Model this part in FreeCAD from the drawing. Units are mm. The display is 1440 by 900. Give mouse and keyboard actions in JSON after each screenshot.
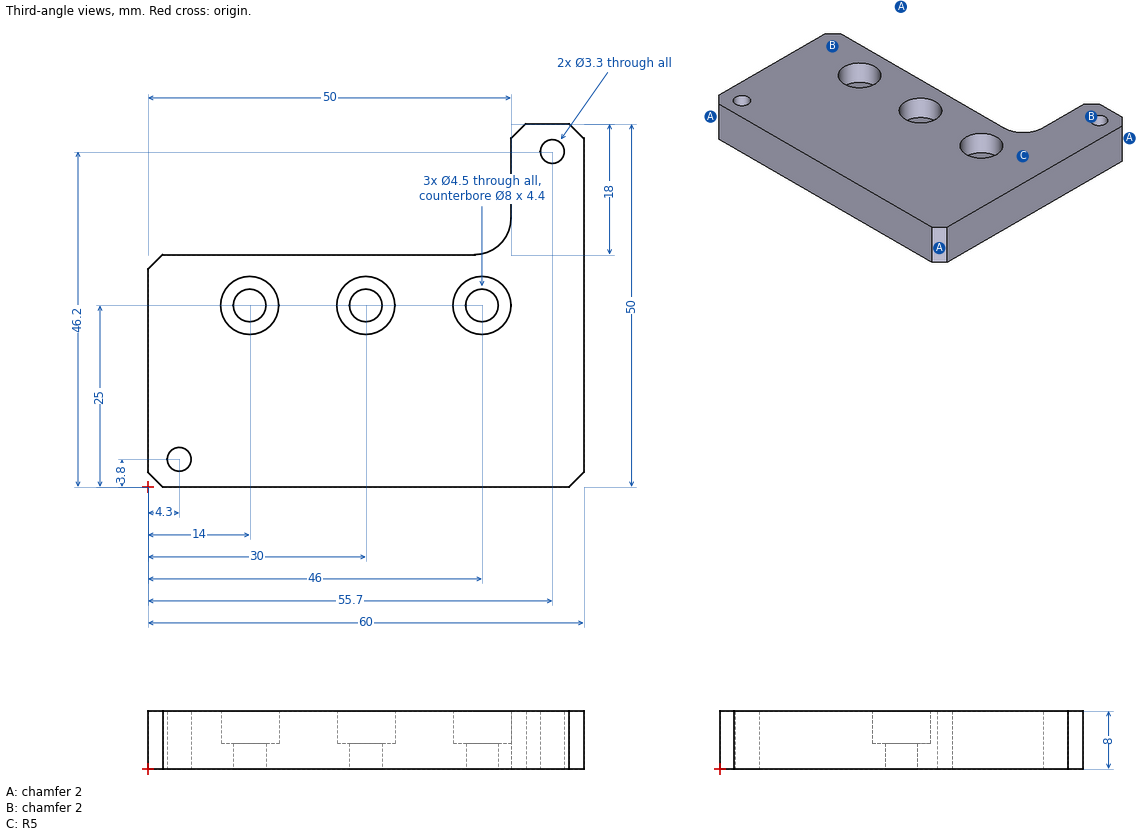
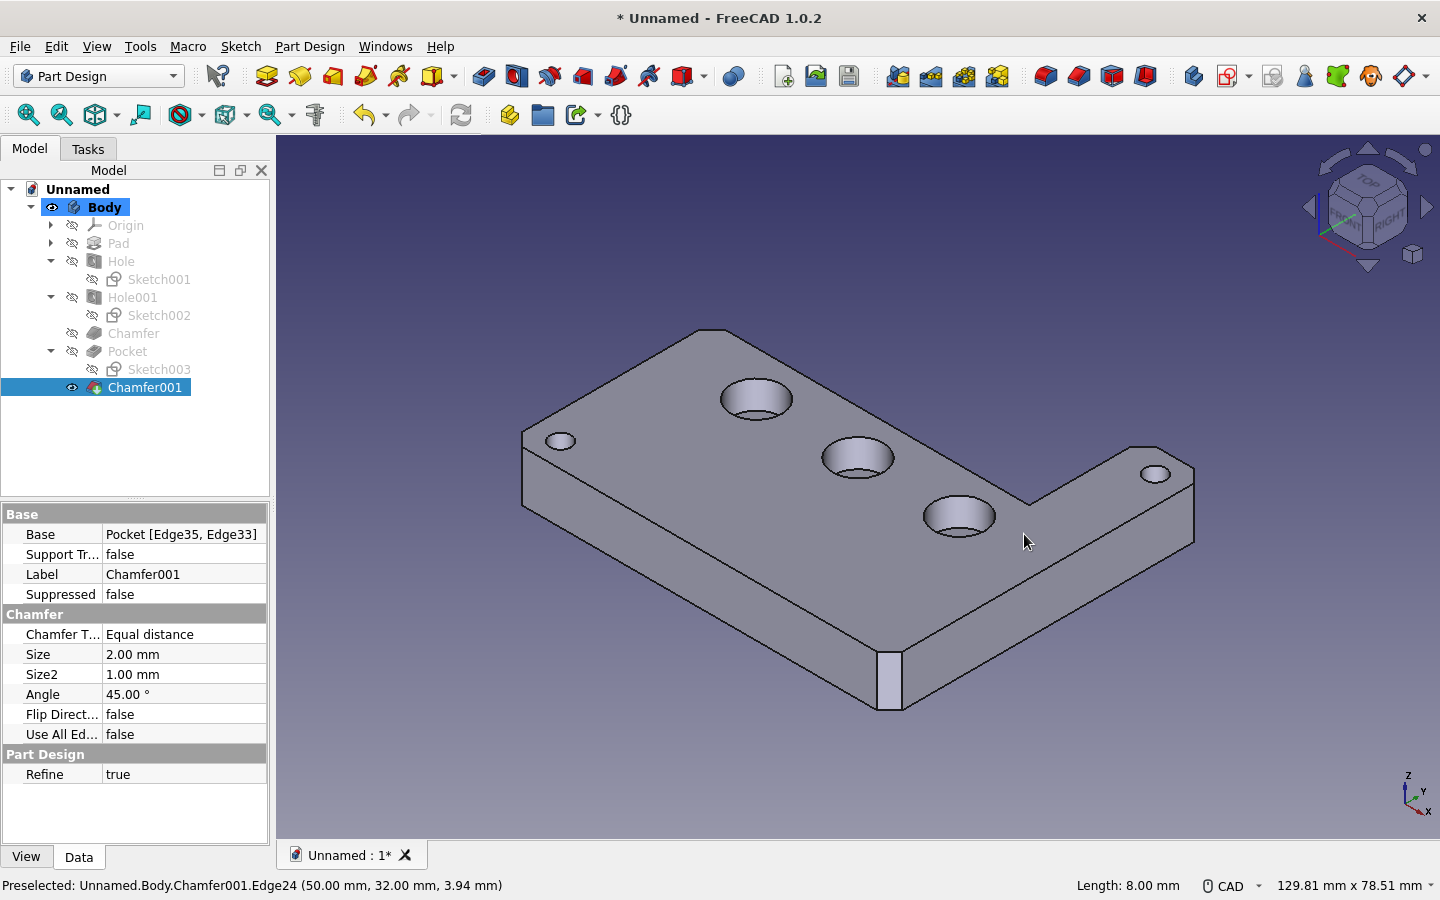
{"action": "left_click", "coordinate": [1046, 76]}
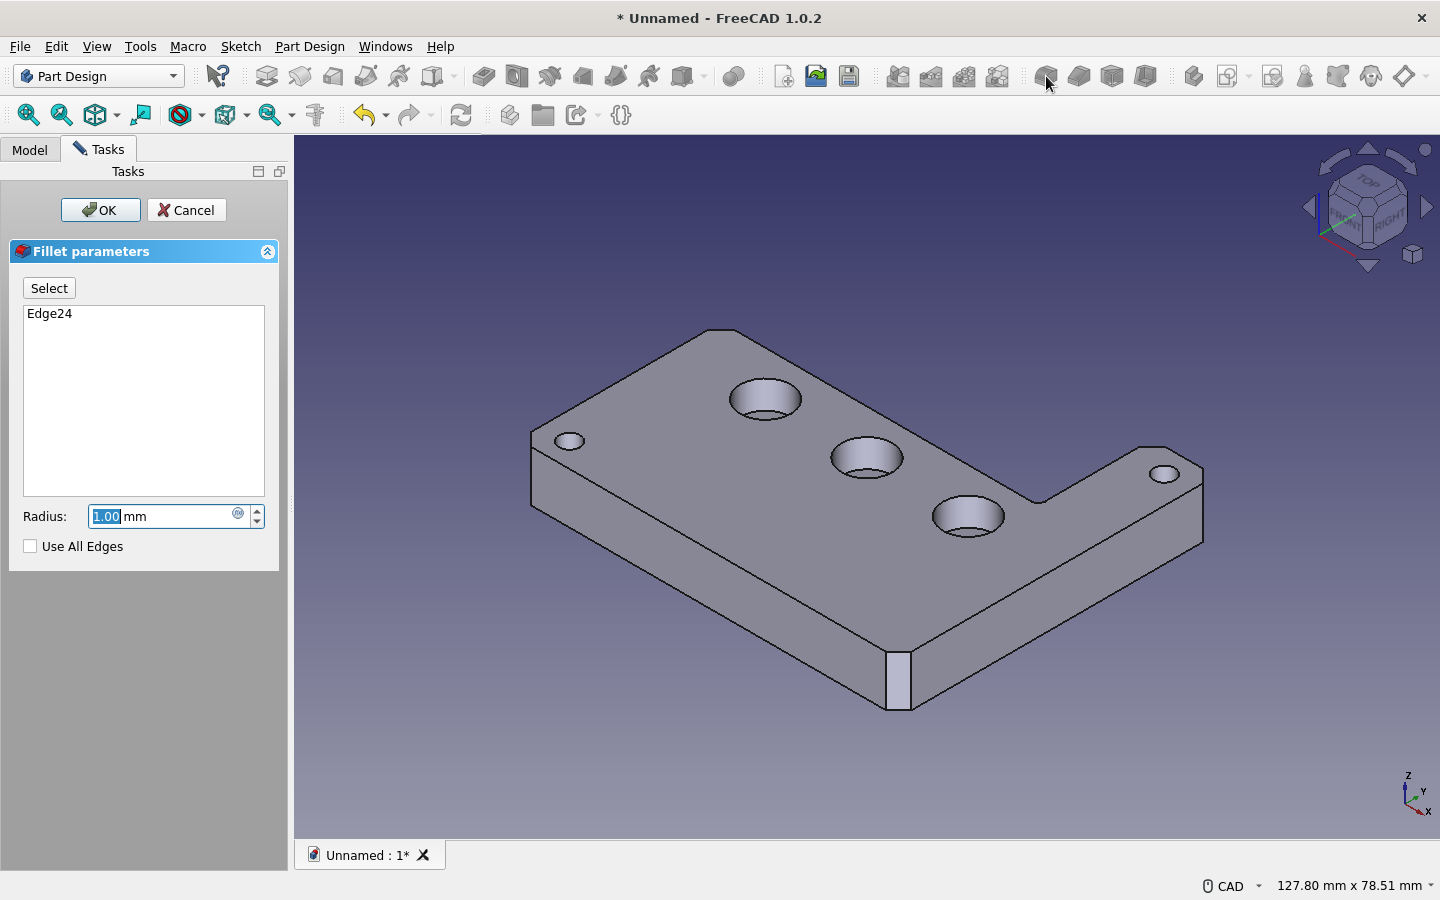
{"action": "type", "text": "5"}
{"action": "key", "text": "Tab"}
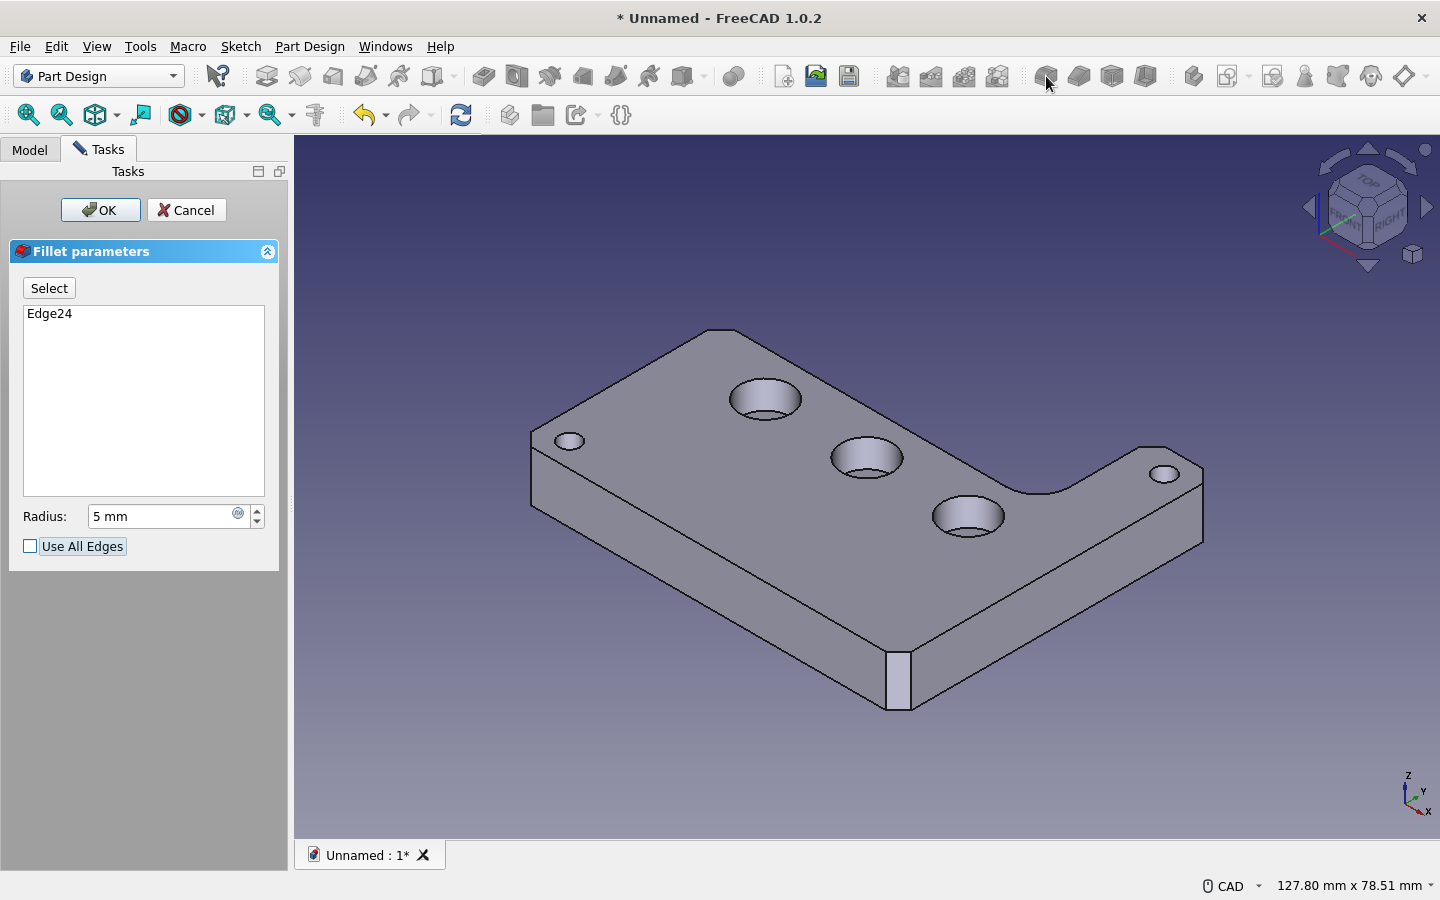
{"action": "left_click", "coordinate": [101, 210]}